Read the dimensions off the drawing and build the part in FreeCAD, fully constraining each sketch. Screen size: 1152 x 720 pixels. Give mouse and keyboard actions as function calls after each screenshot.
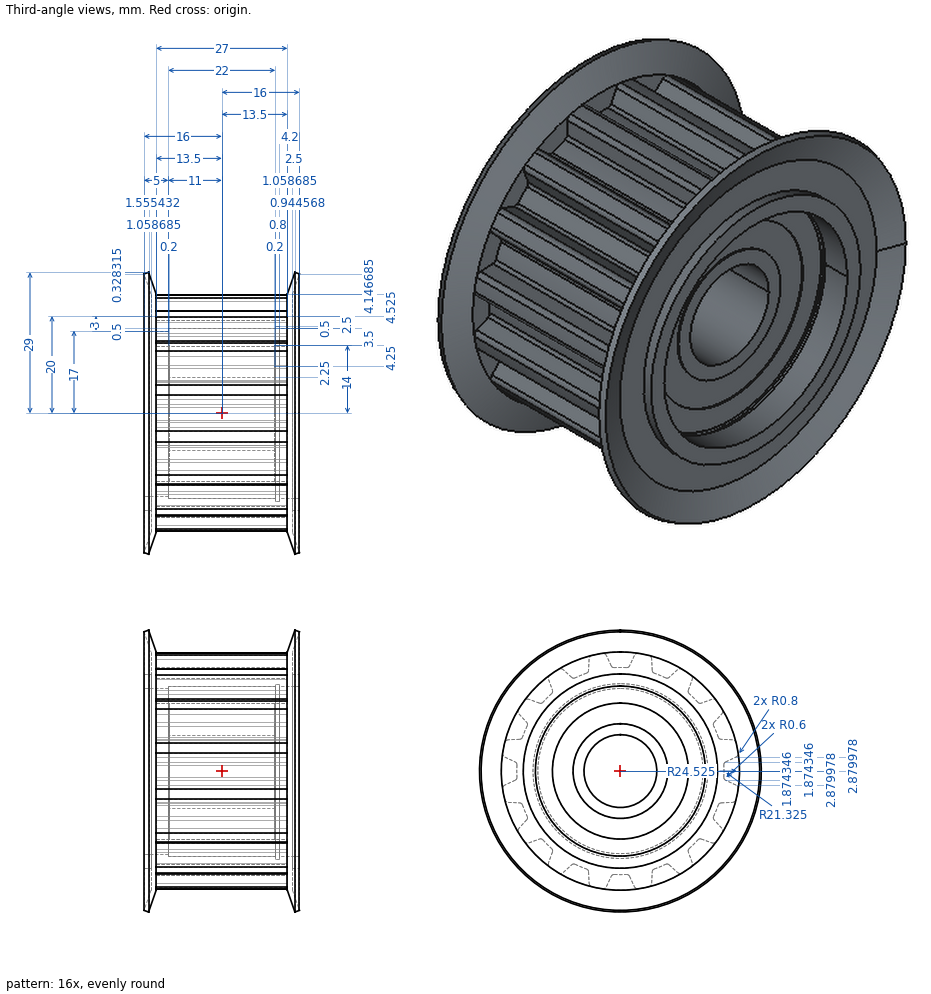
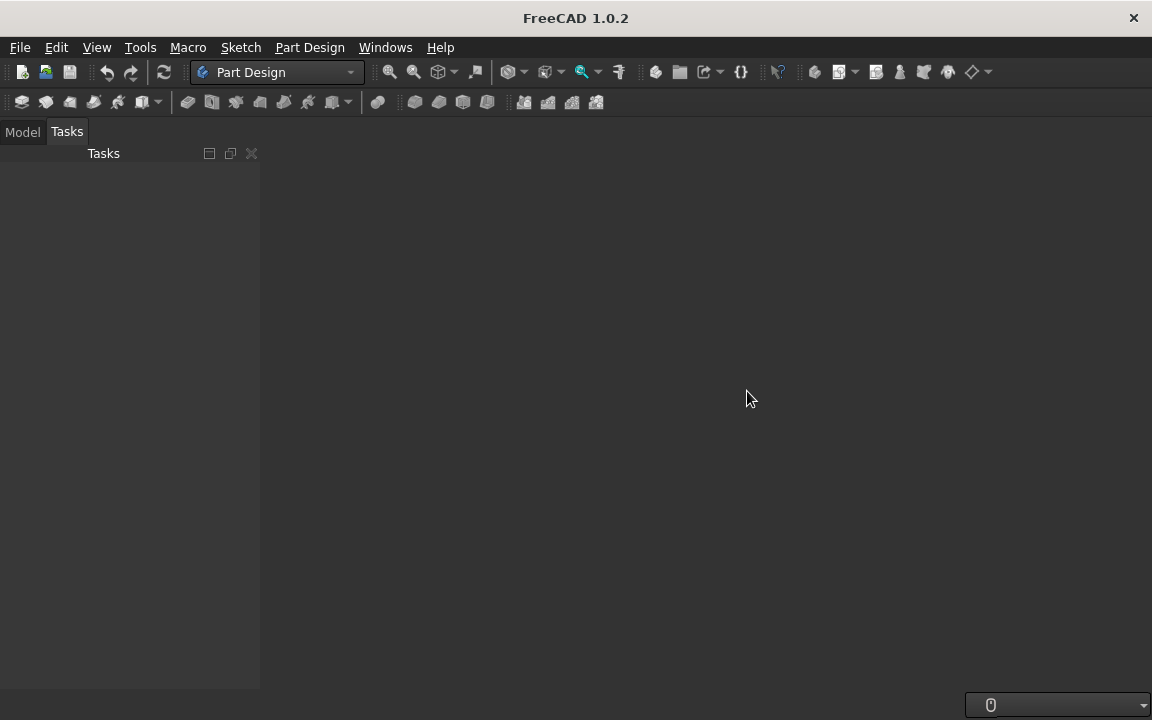
click(22, 72)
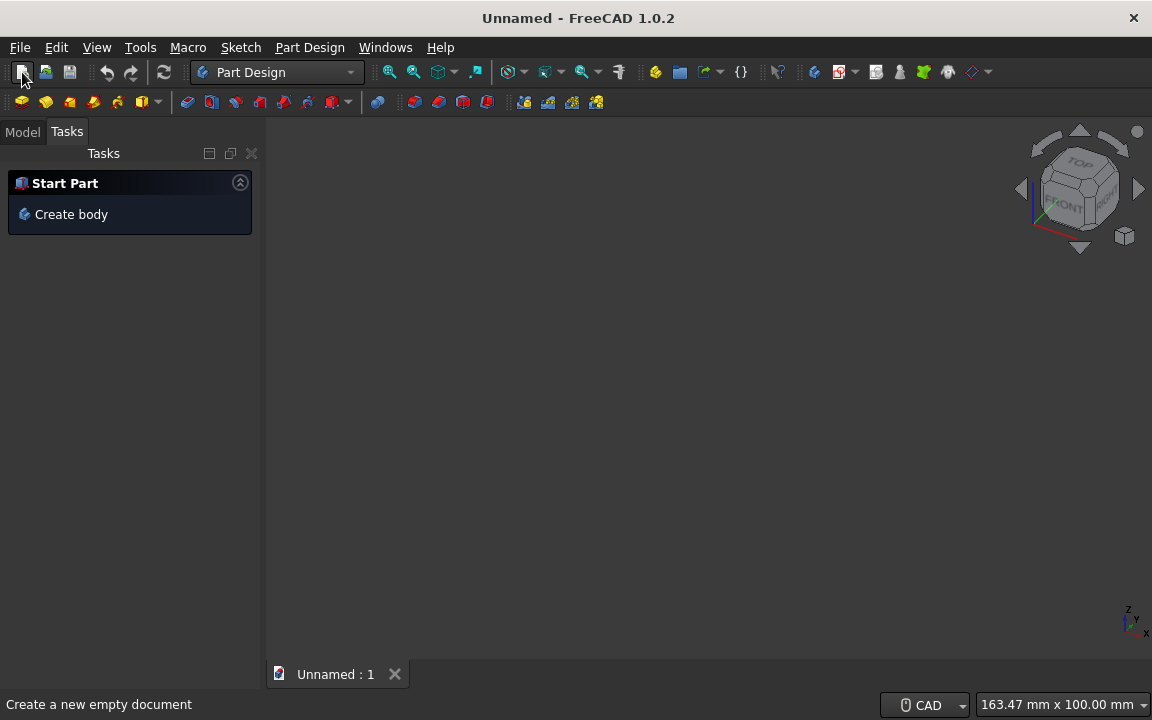
click(840, 72)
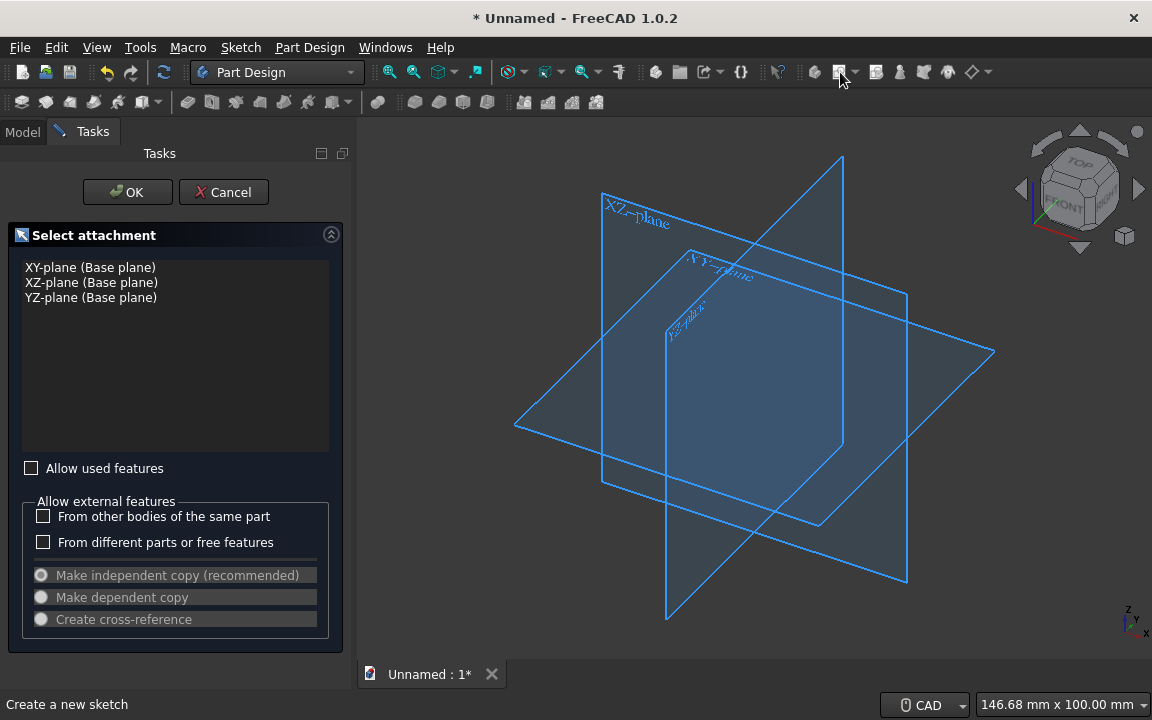
click(82, 268)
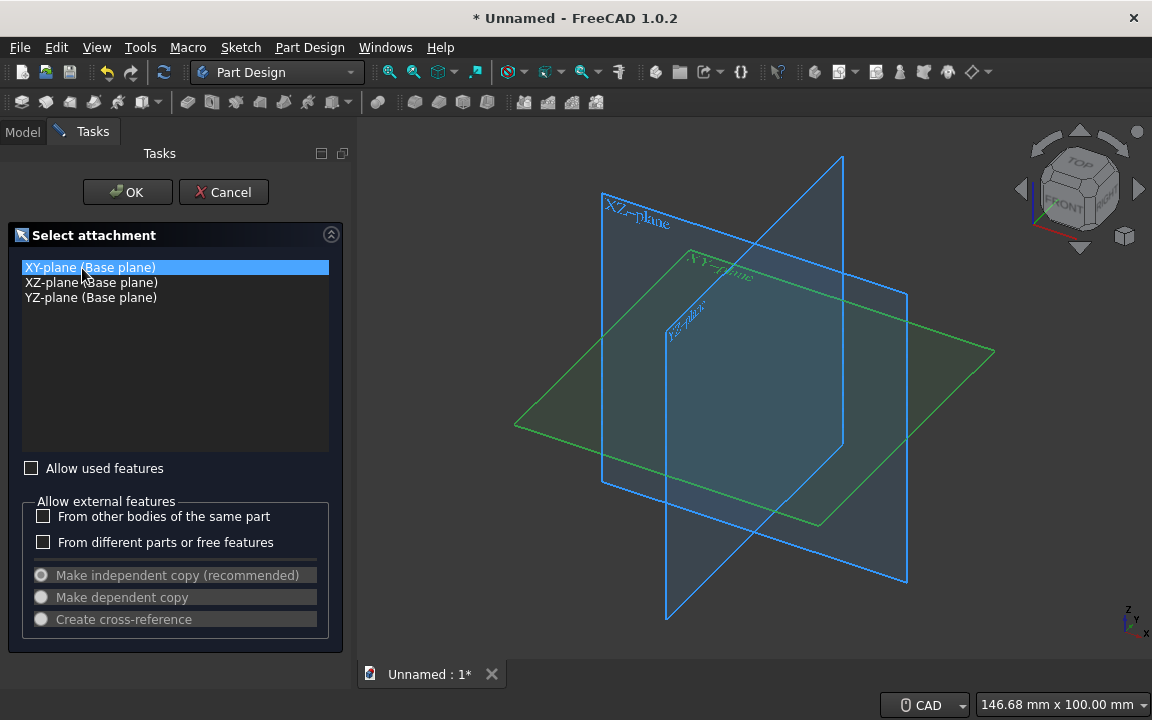
click(128, 192)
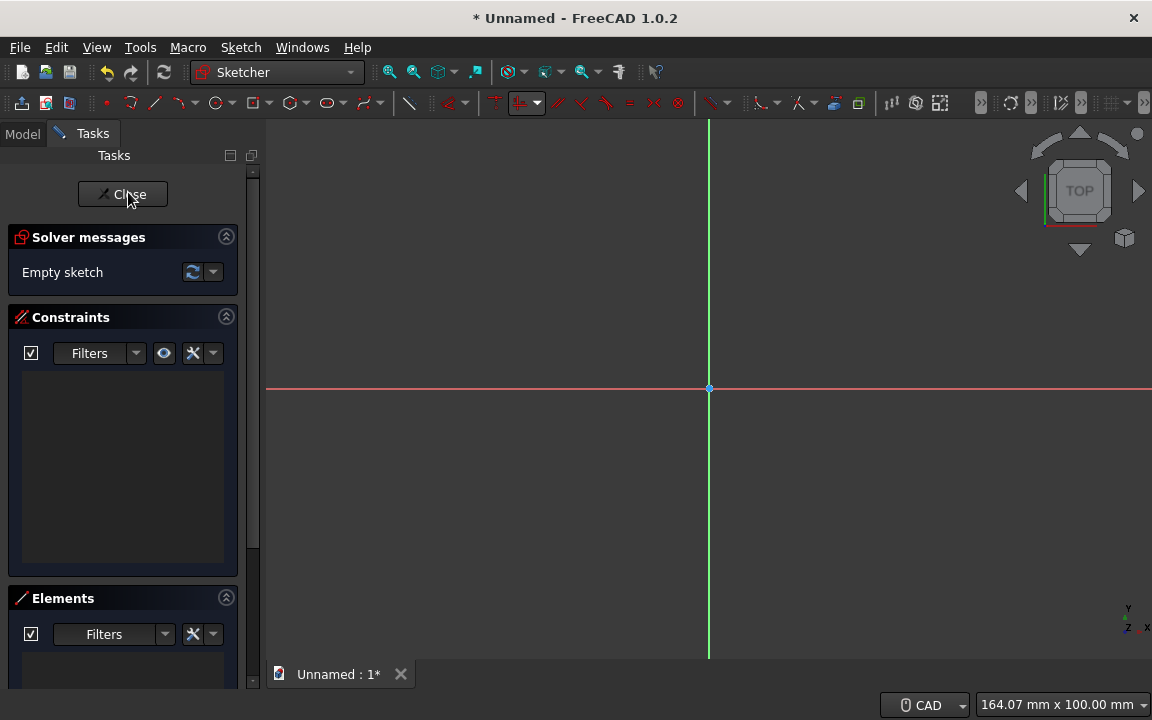
scroll(749, 284, up, 5)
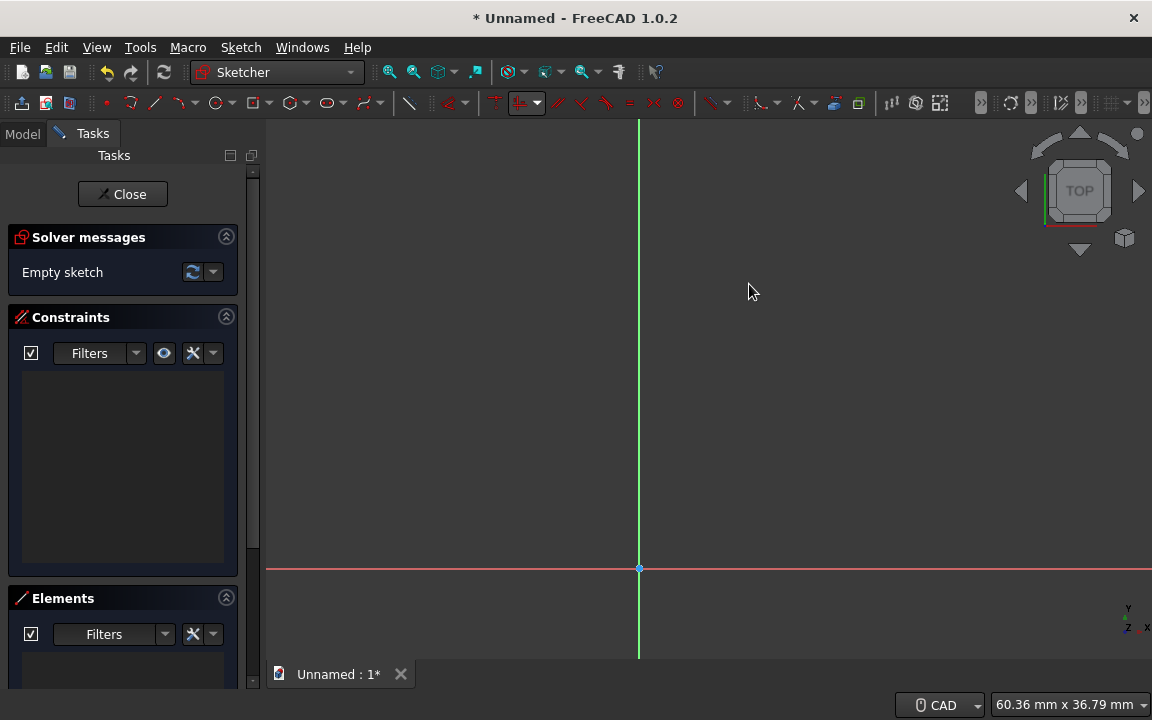
click(132, 104)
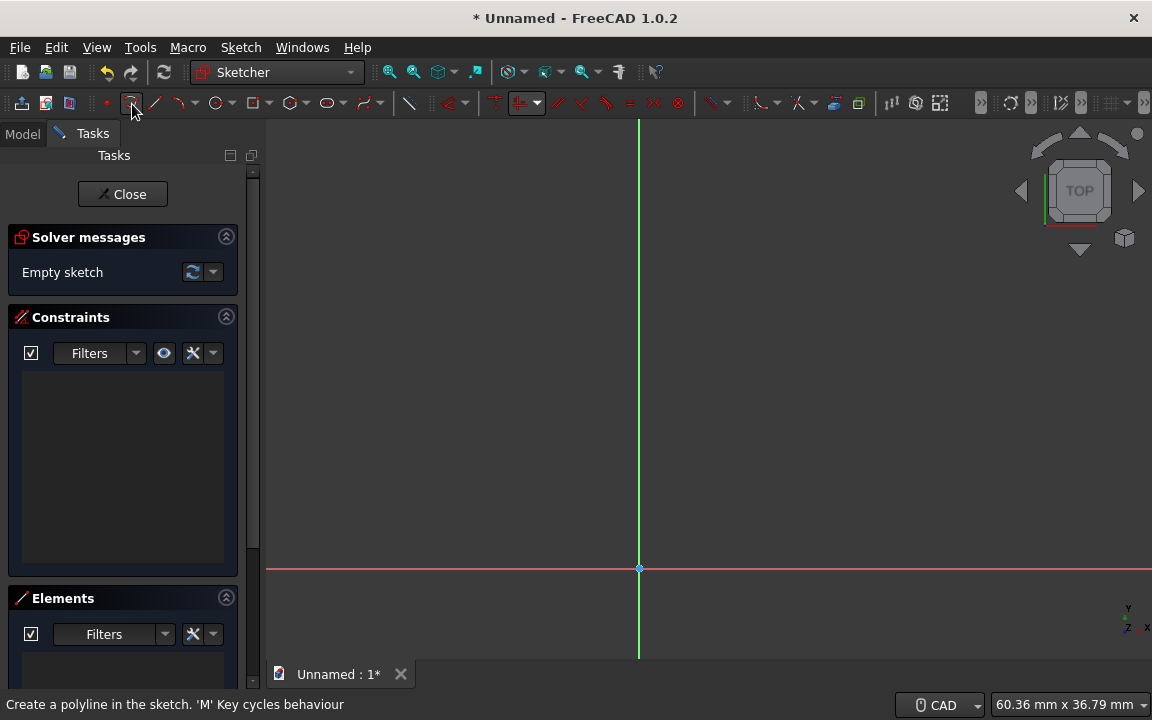
click(478, 319)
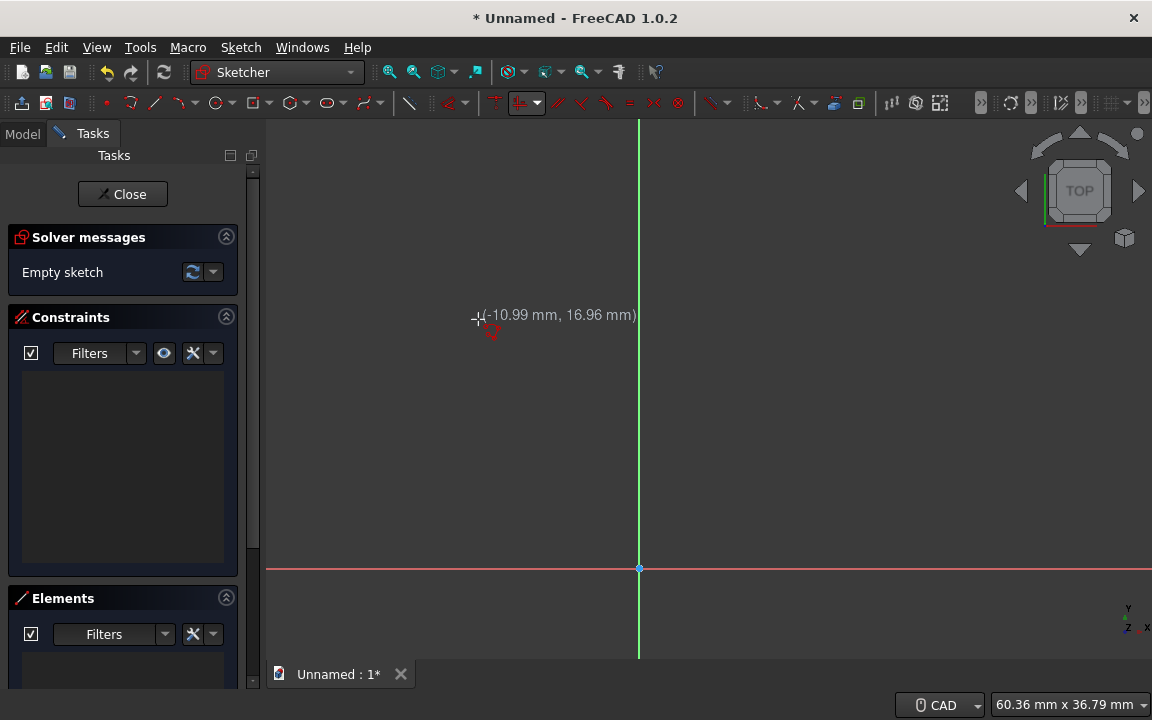
scroll(478, 312, up, 4)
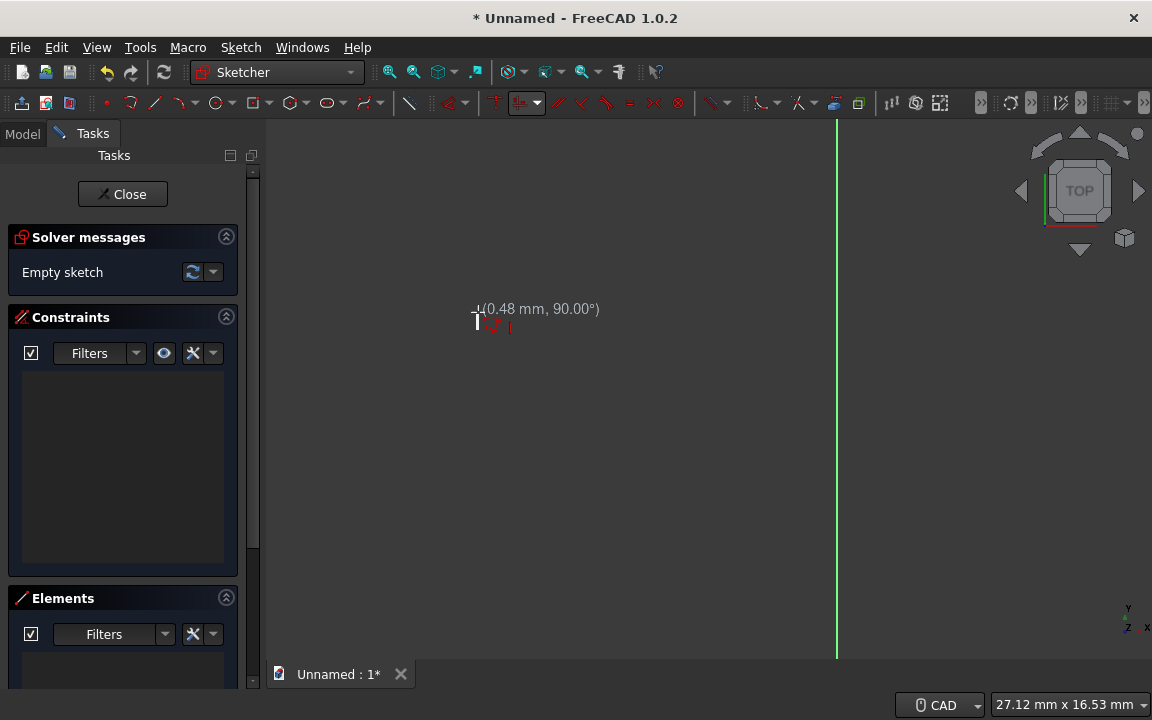
click(478, 312)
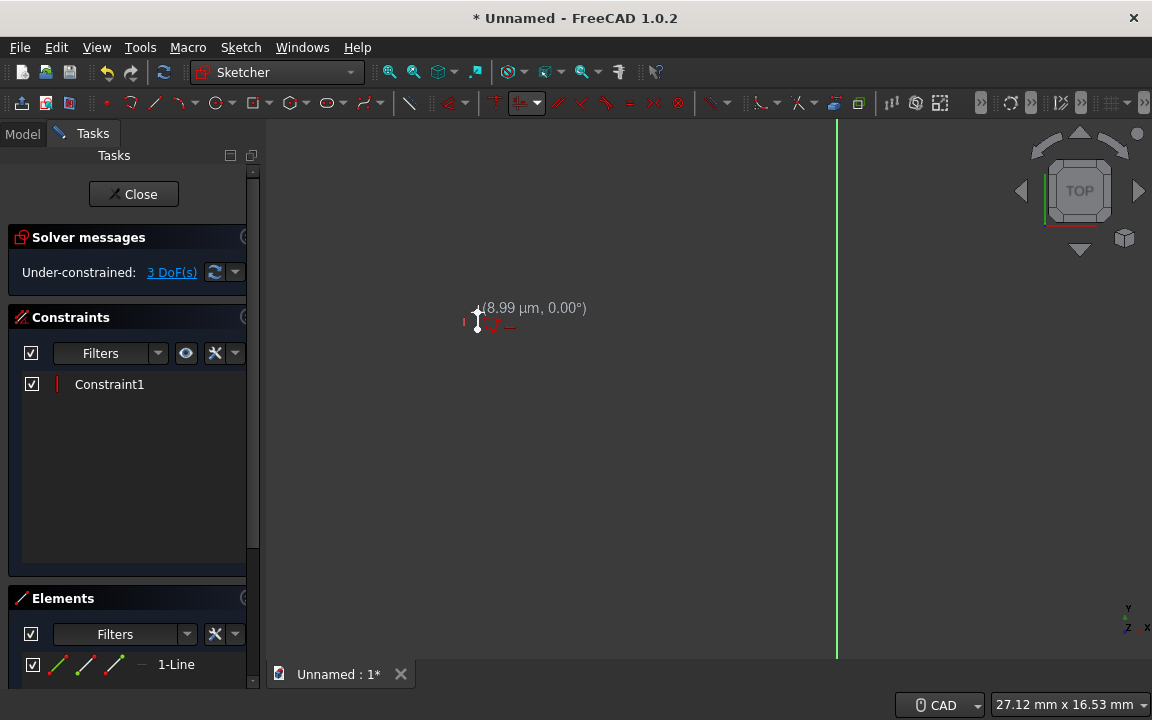
scroll(480, 313, down, 4)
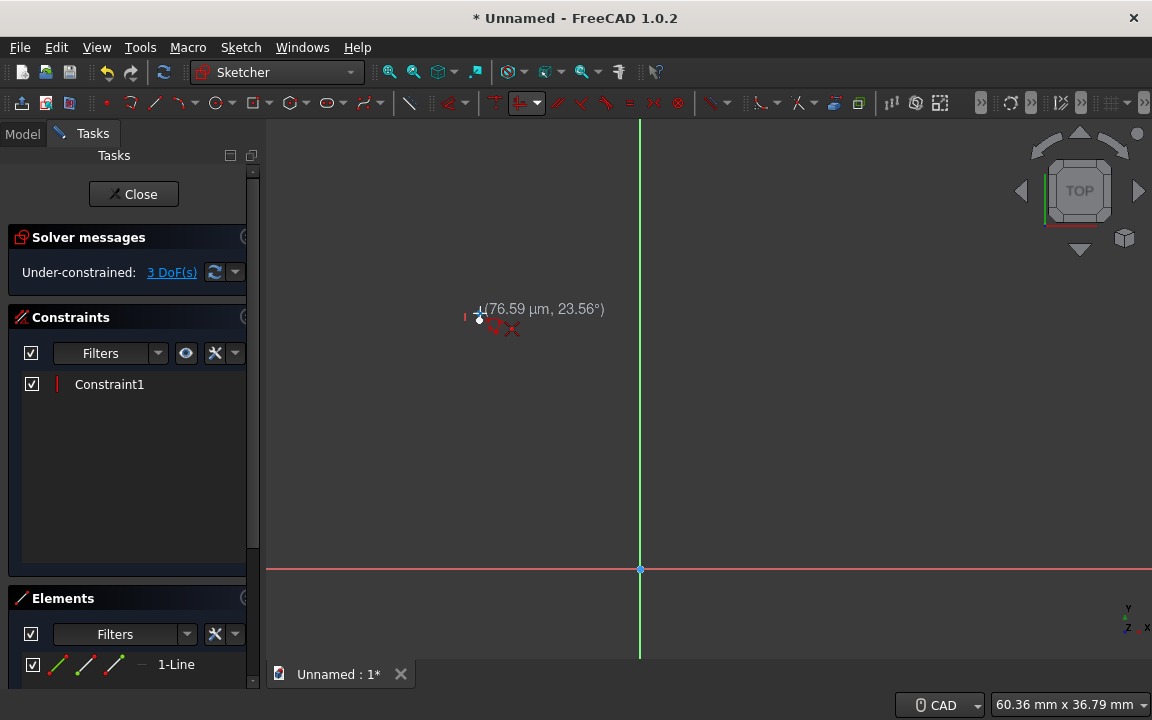
click(802, 313)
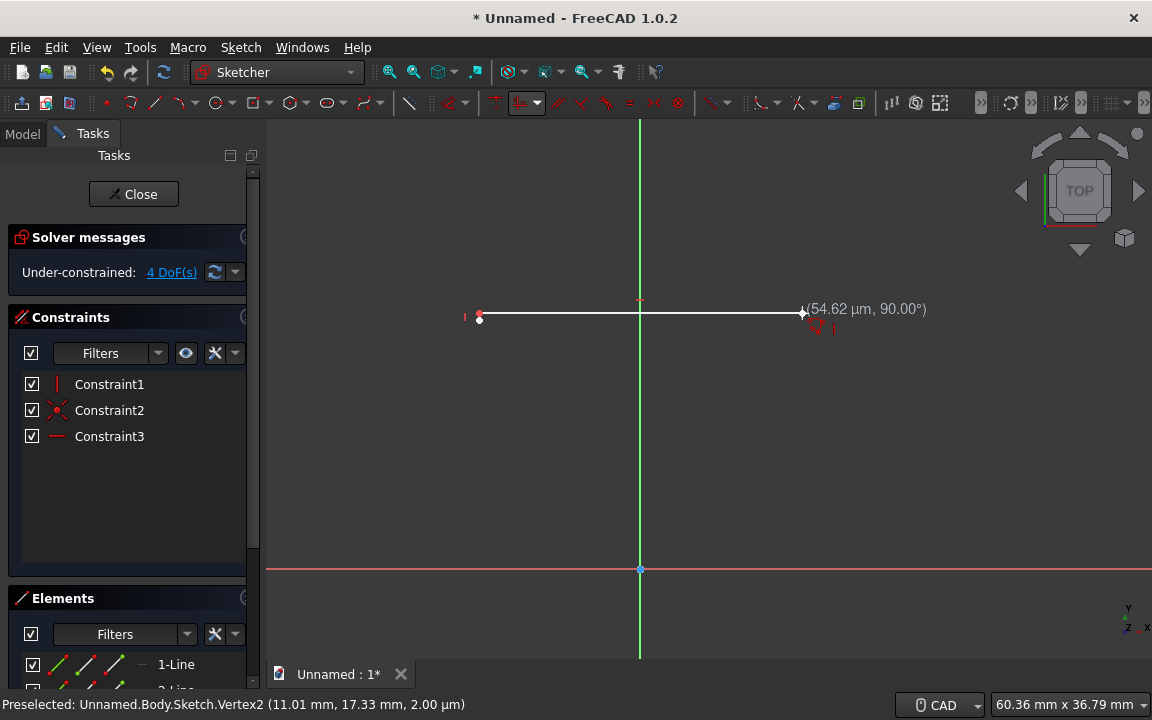
scroll(802, 305, up, 4)